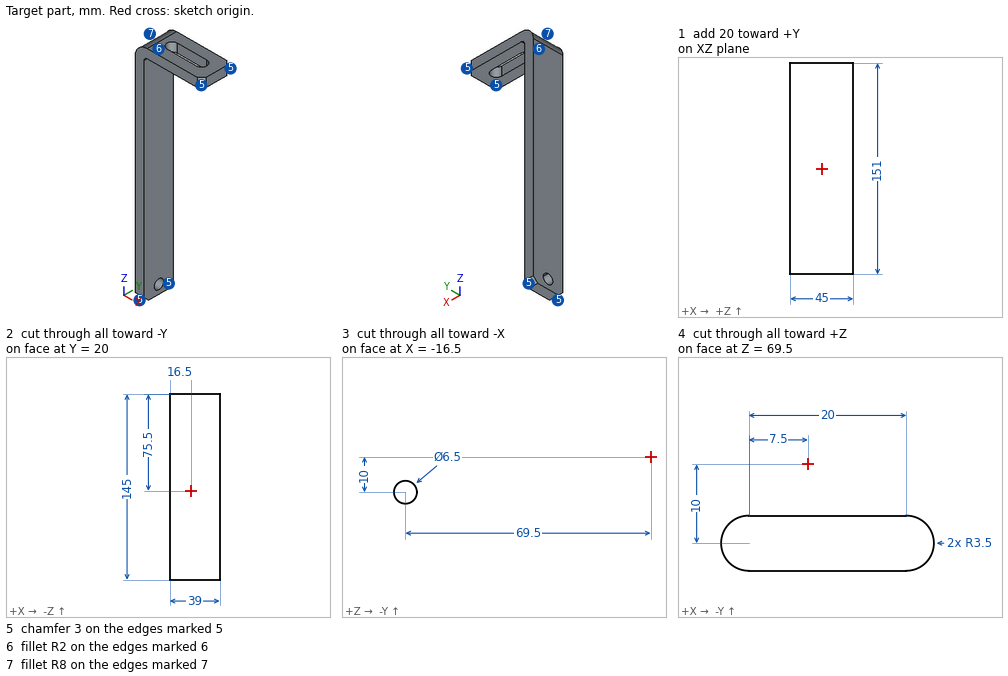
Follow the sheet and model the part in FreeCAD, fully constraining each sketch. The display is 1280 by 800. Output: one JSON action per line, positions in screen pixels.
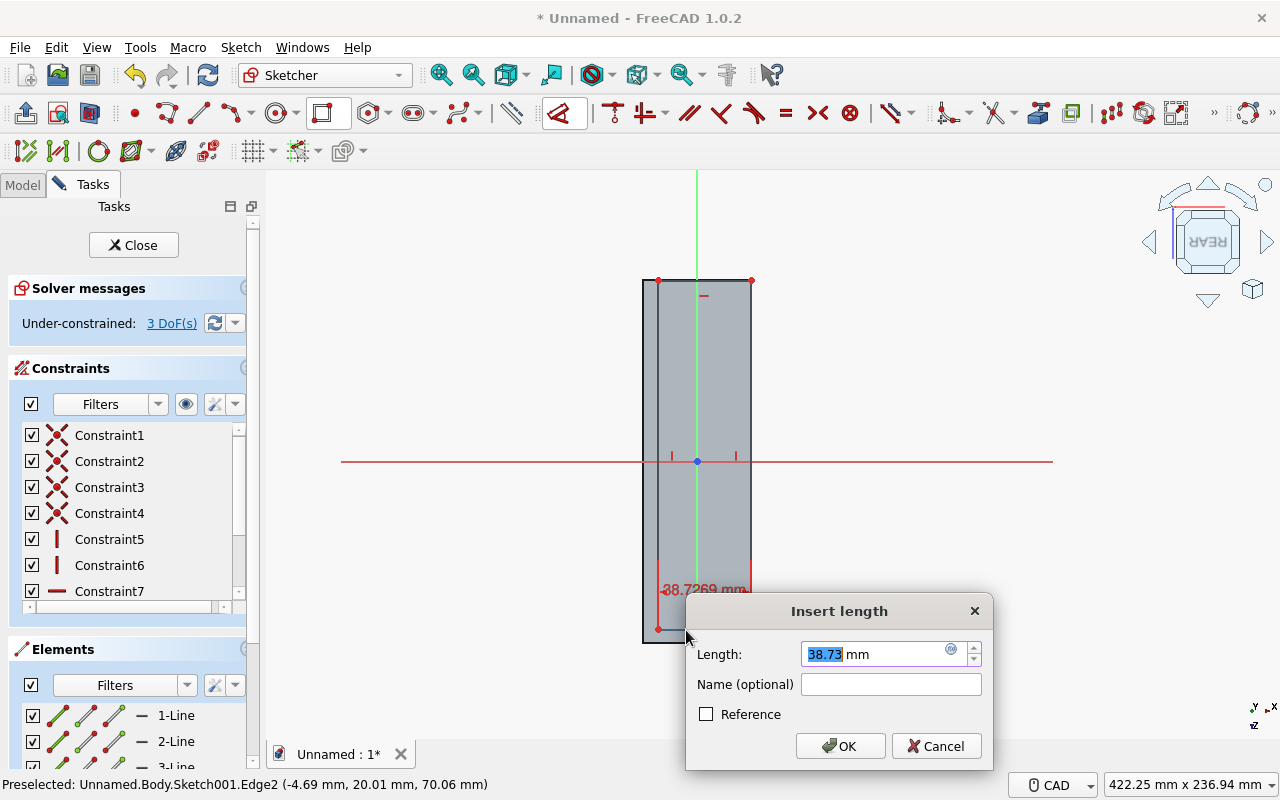
{"action": "type", "text": "39"}
{"action": "key", "text": "Return"}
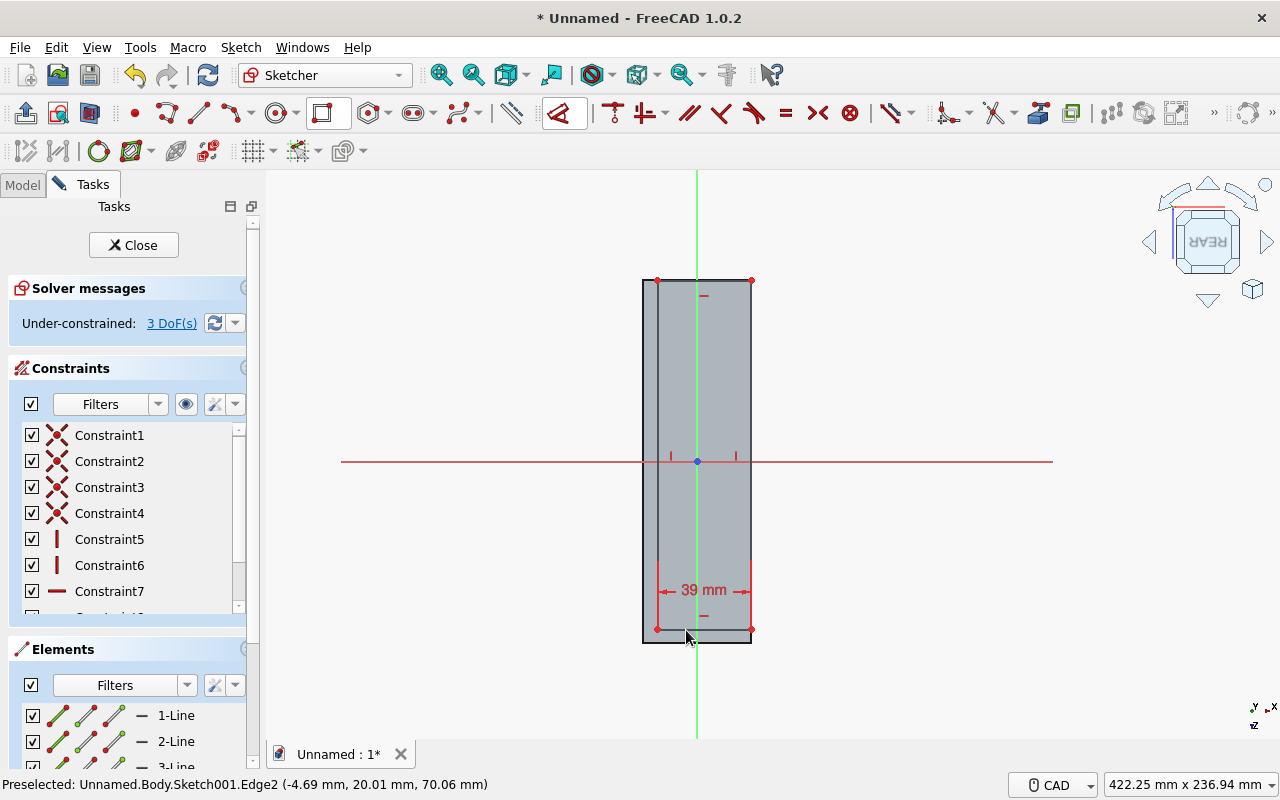
{"action": "left_click", "coordinate": [658, 386]}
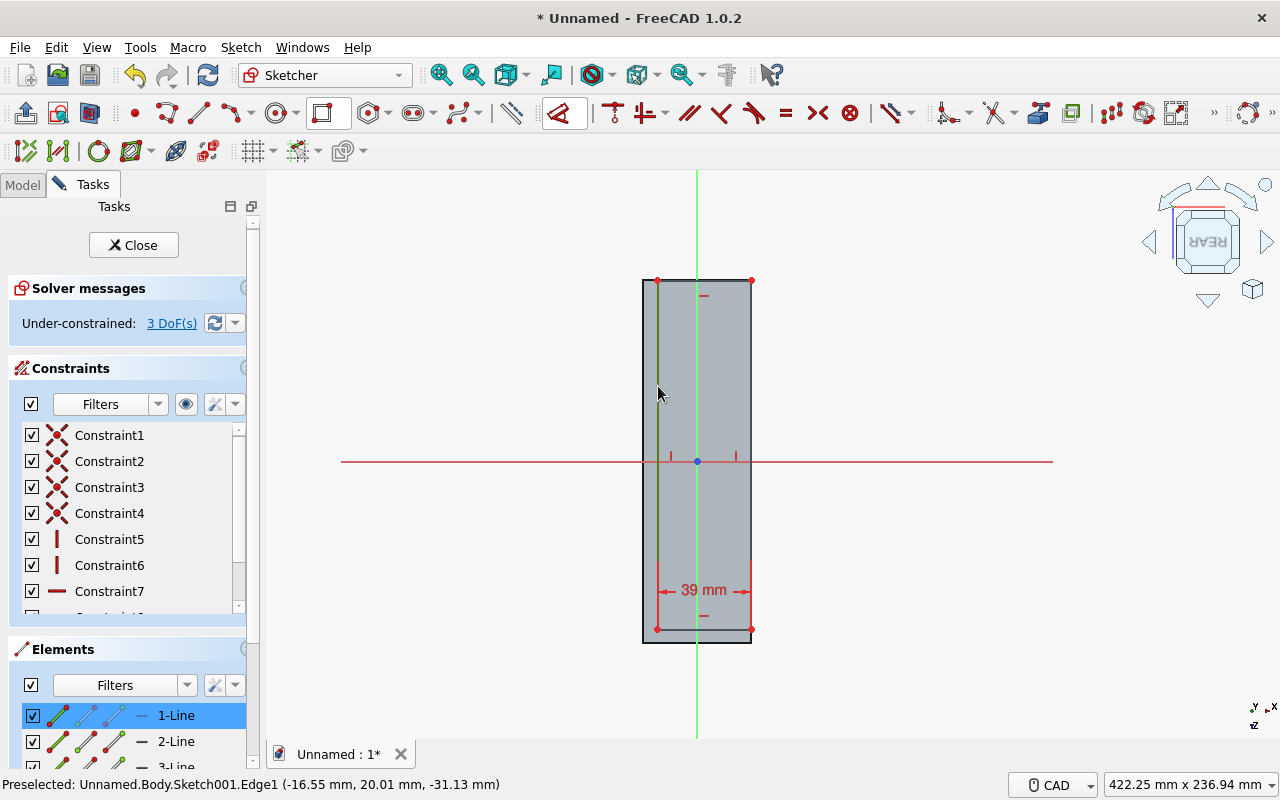
{"action": "key", "text": "i"}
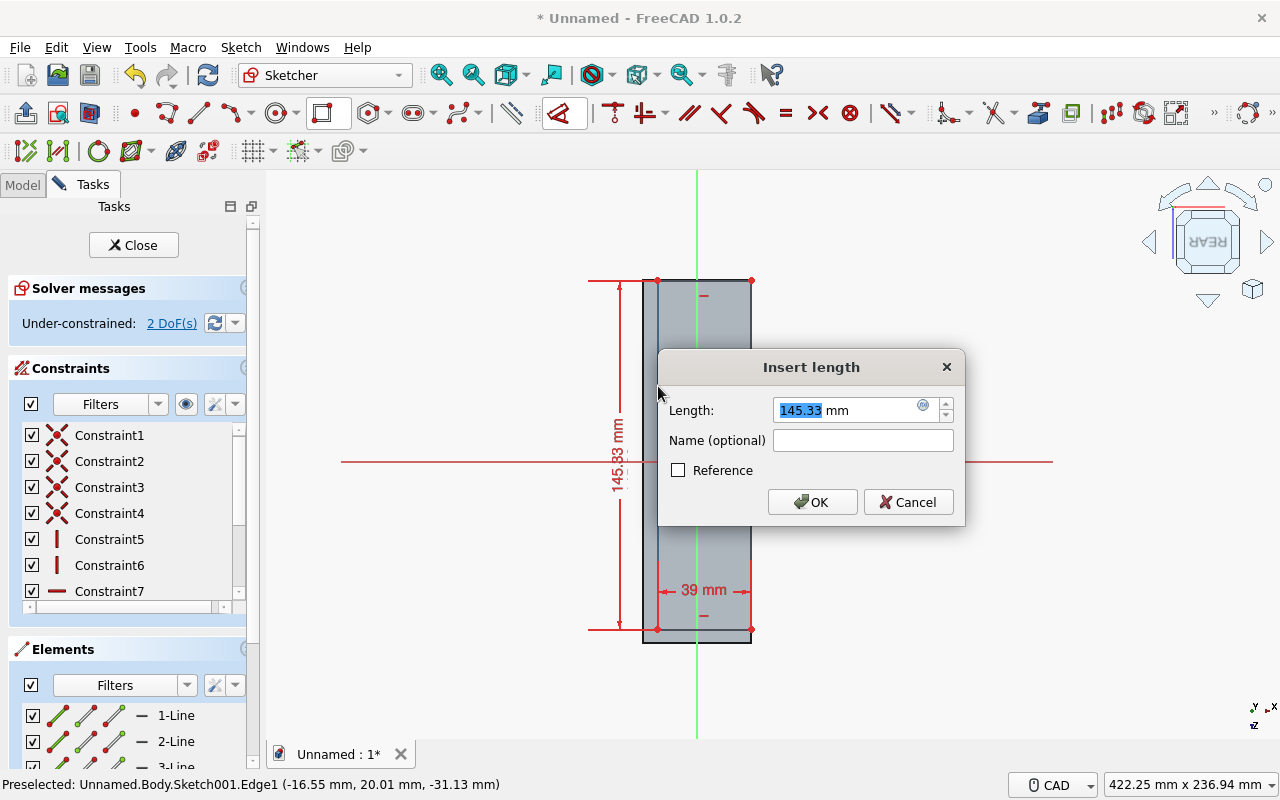
{"action": "type", "text": "145"}
{"action": "key", "text": "Return"}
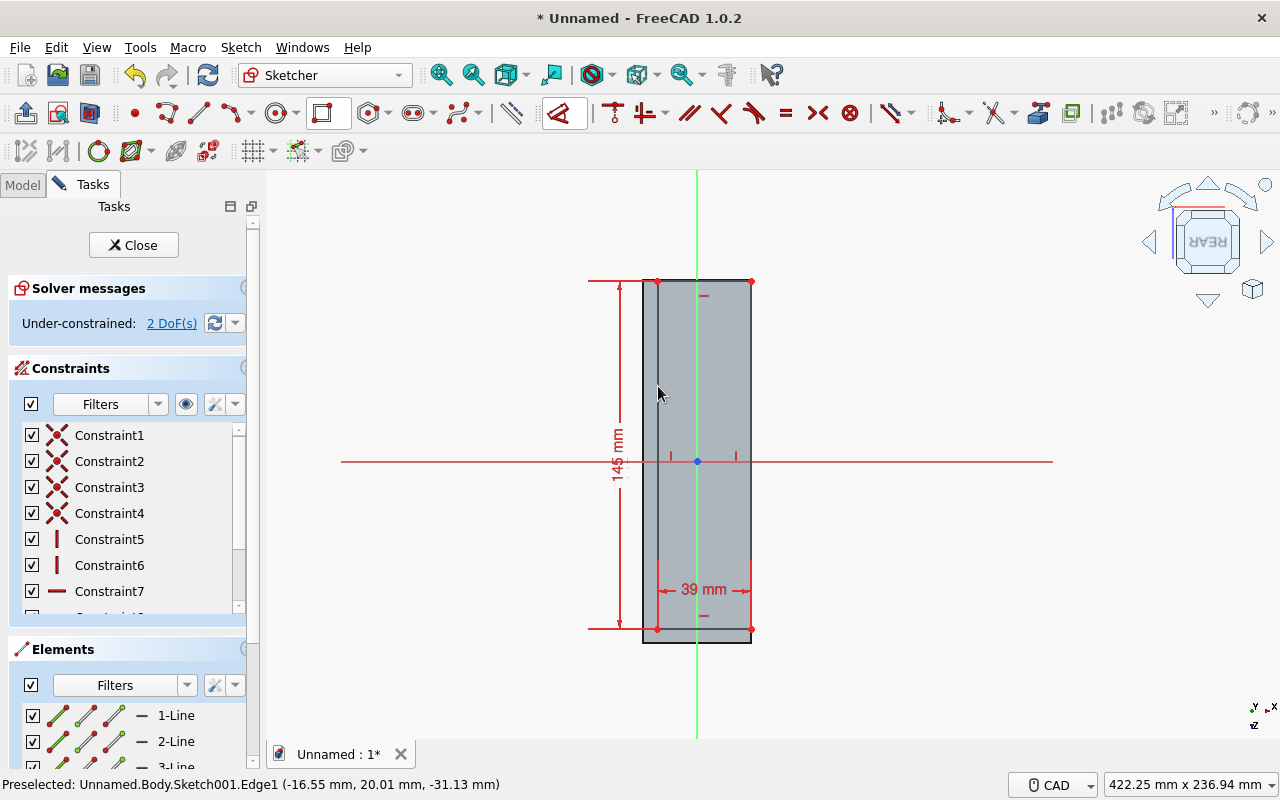
{"action": "left_click", "coordinate": [658, 281]}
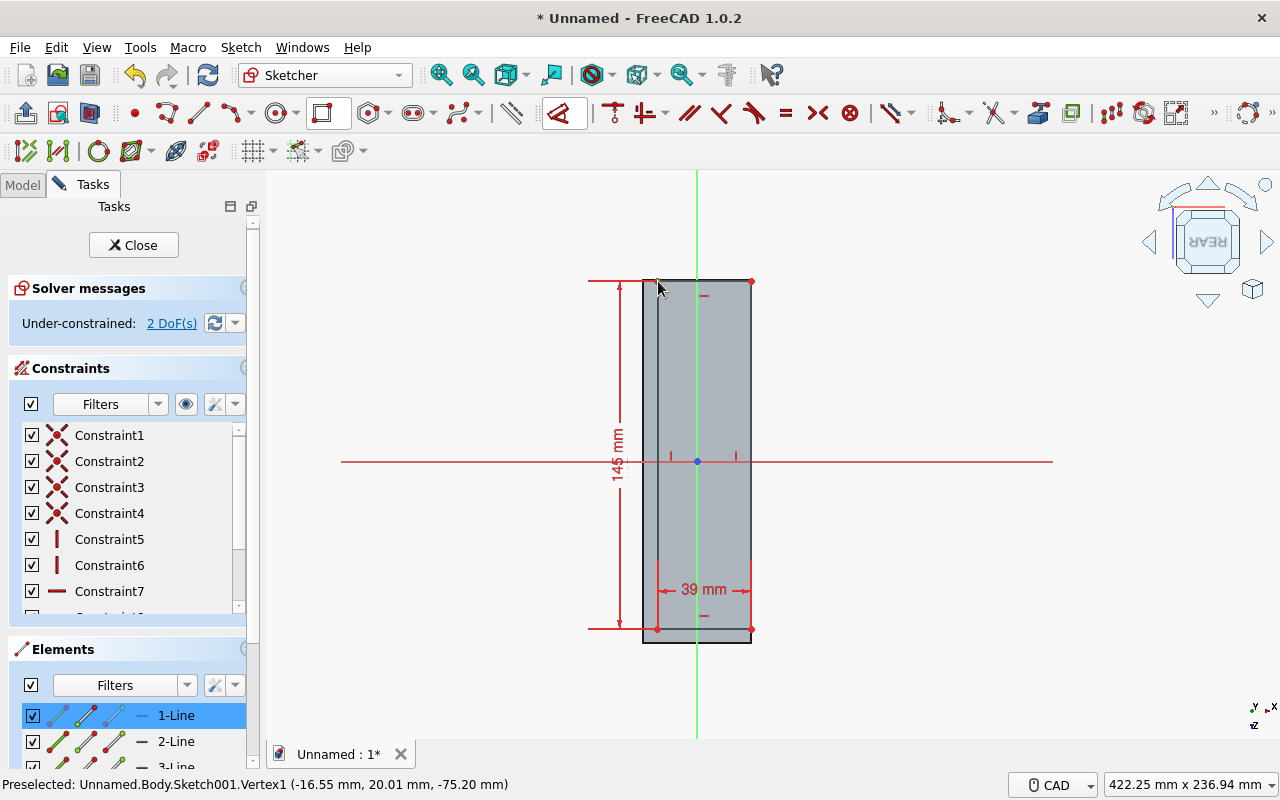
{"action": "key", "text": "l"}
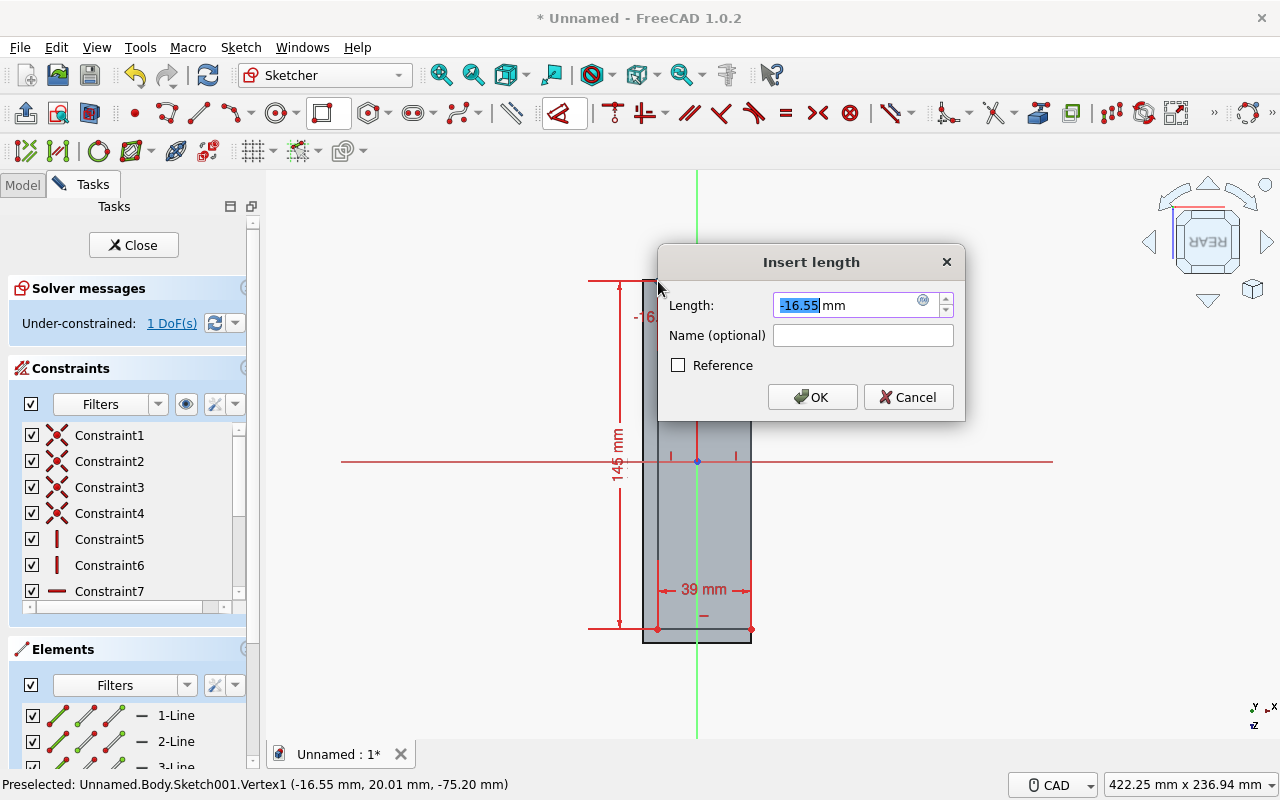
{"action": "type", "text": "-16.5"}
{"action": "key", "text": "Return"}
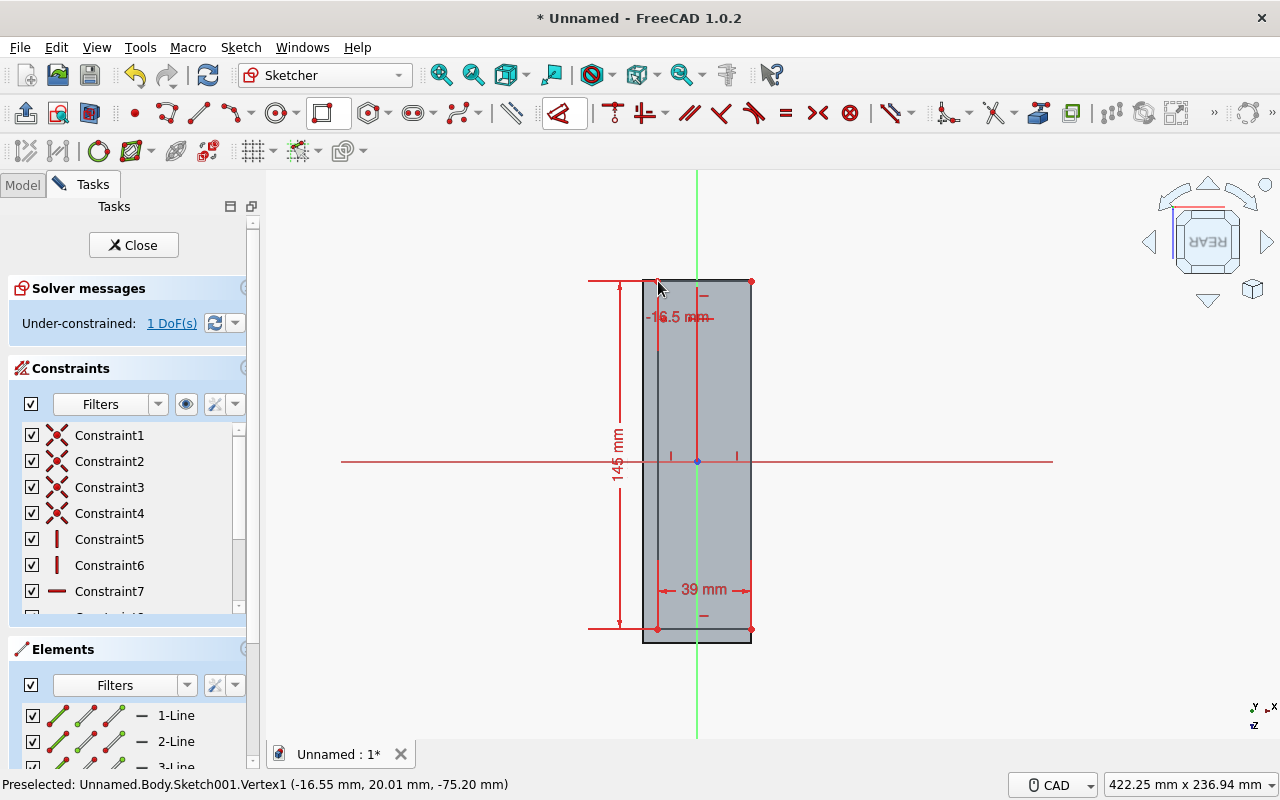
{"action": "left_click", "coordinate": [658, 281]}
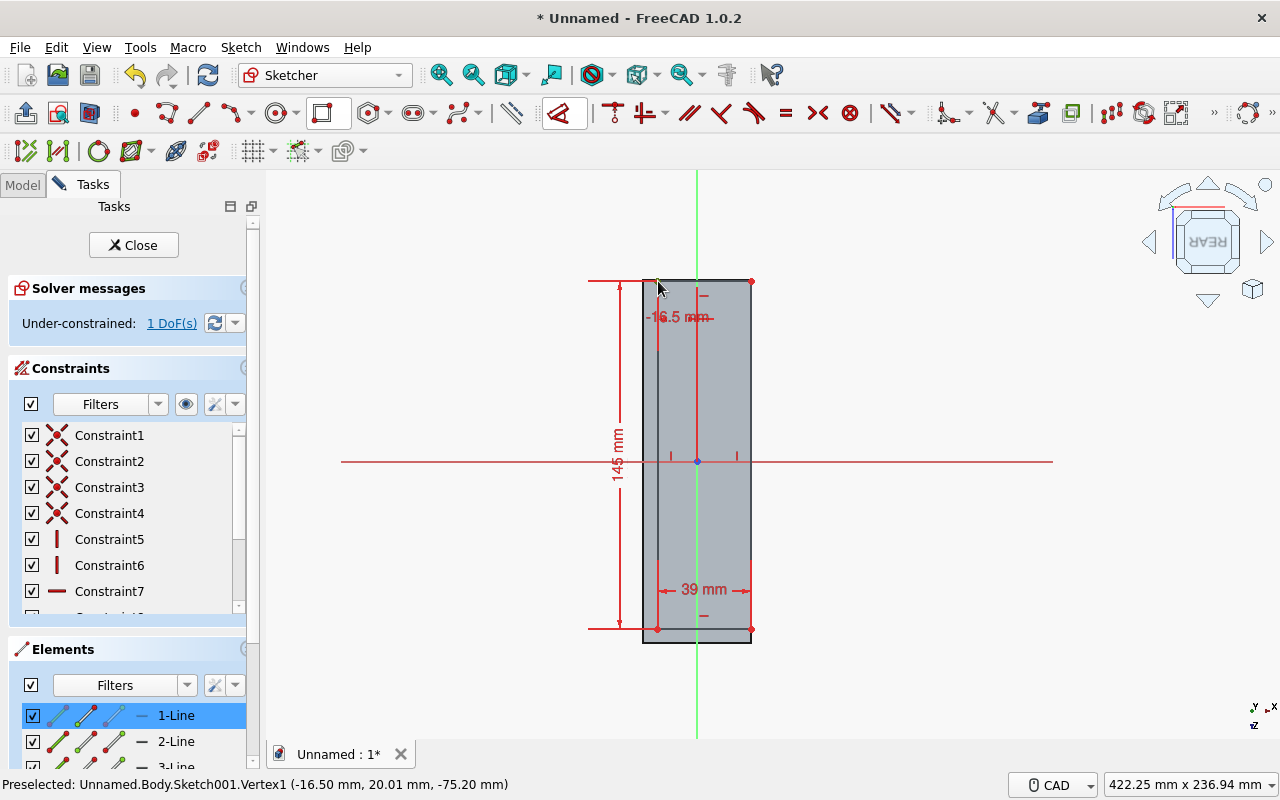
{"action": "left_click", "coordinate": [582, 114]}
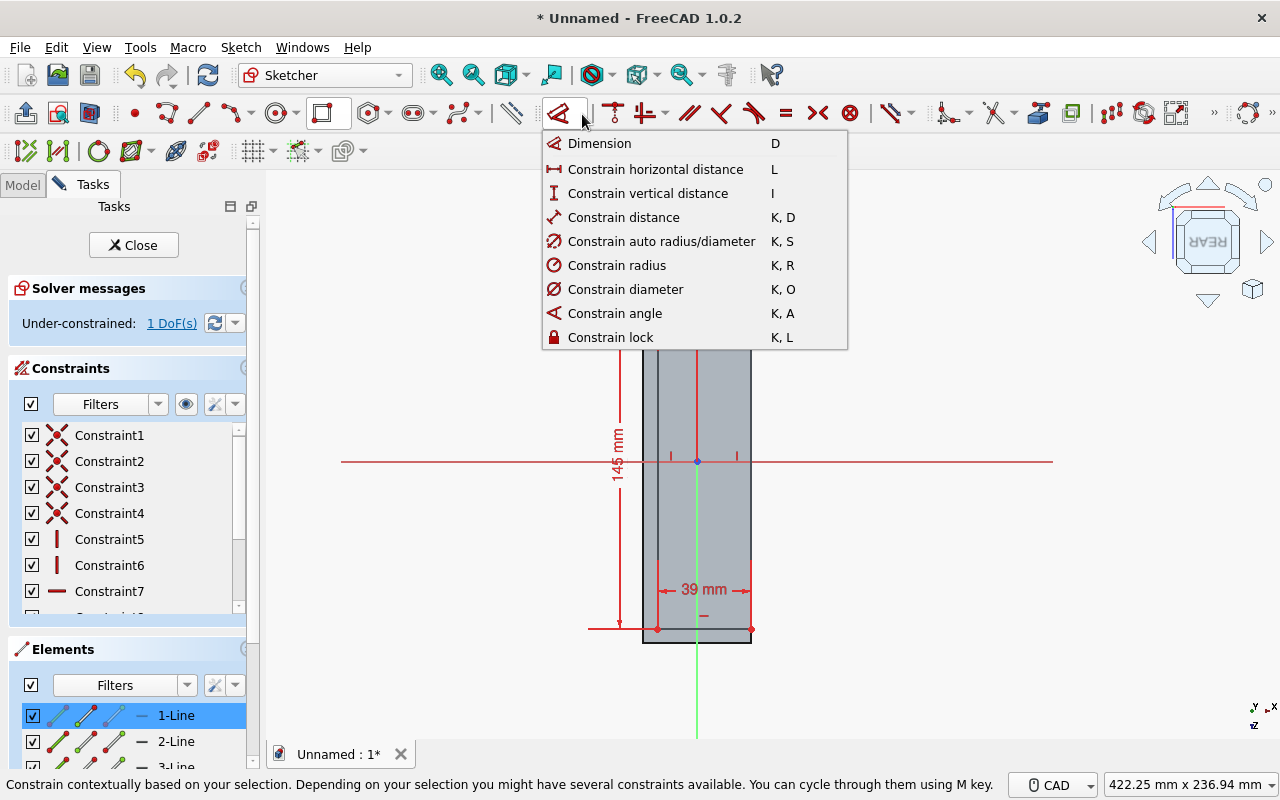
{"action": "left_click", "coordinate": [695, 193]}